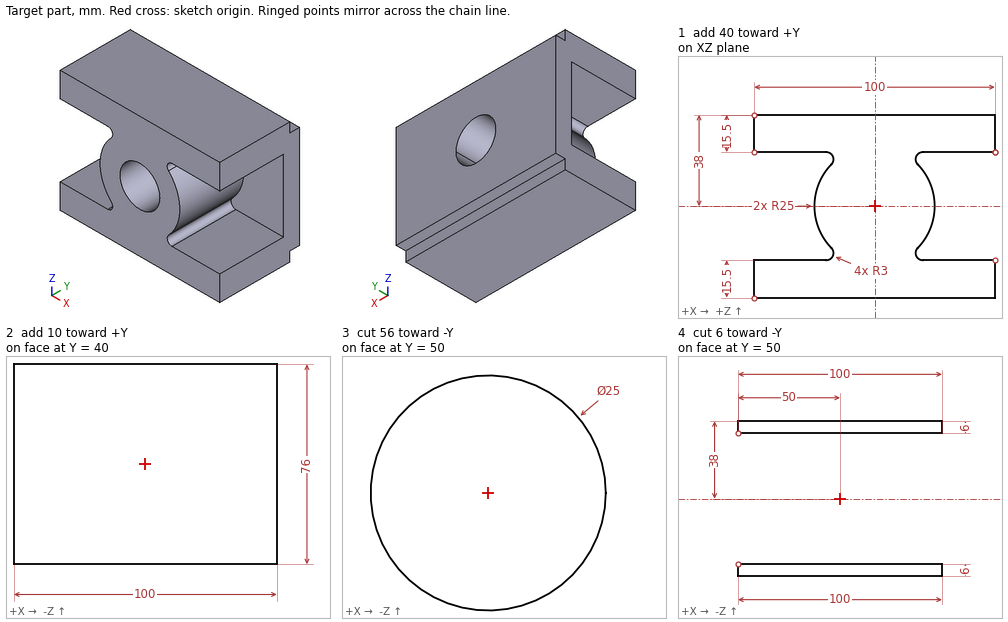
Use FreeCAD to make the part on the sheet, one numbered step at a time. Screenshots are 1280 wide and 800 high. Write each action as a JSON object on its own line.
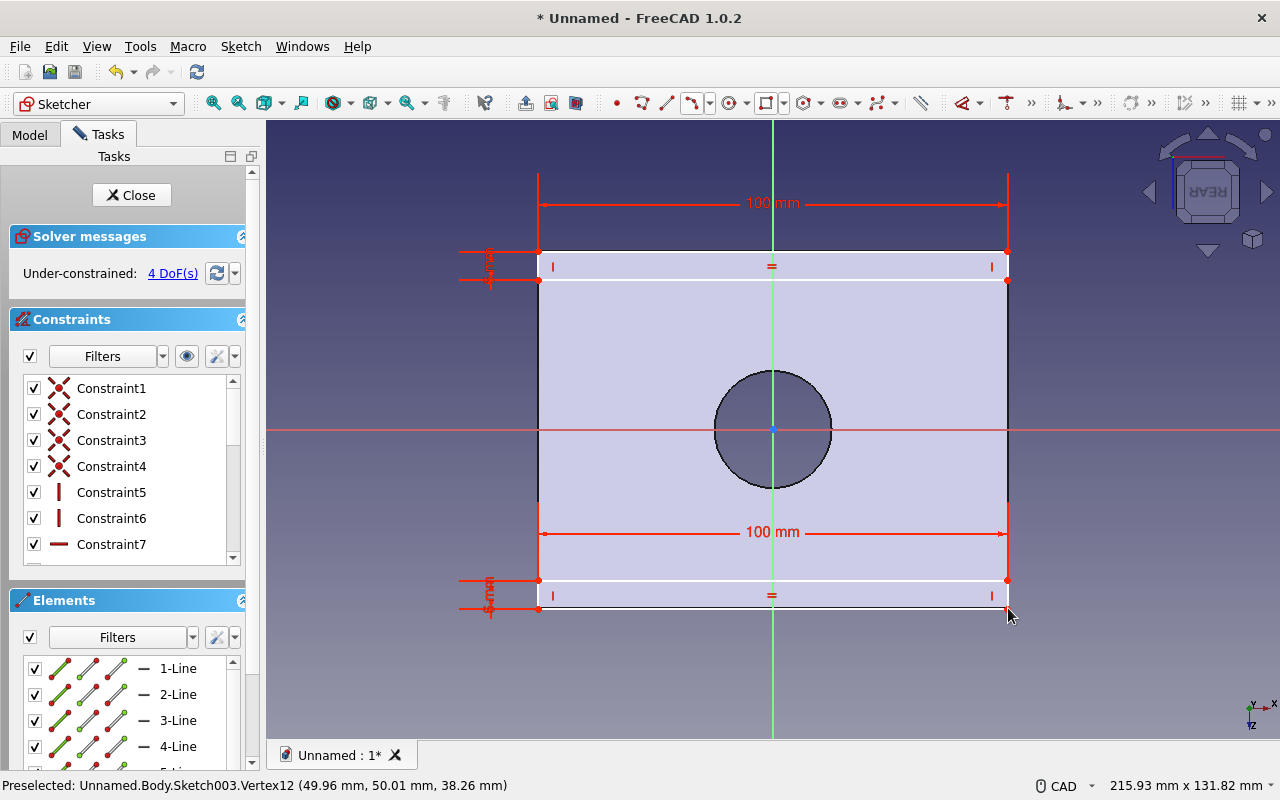
{"action": "left_click", "coordinate": [538, 280]}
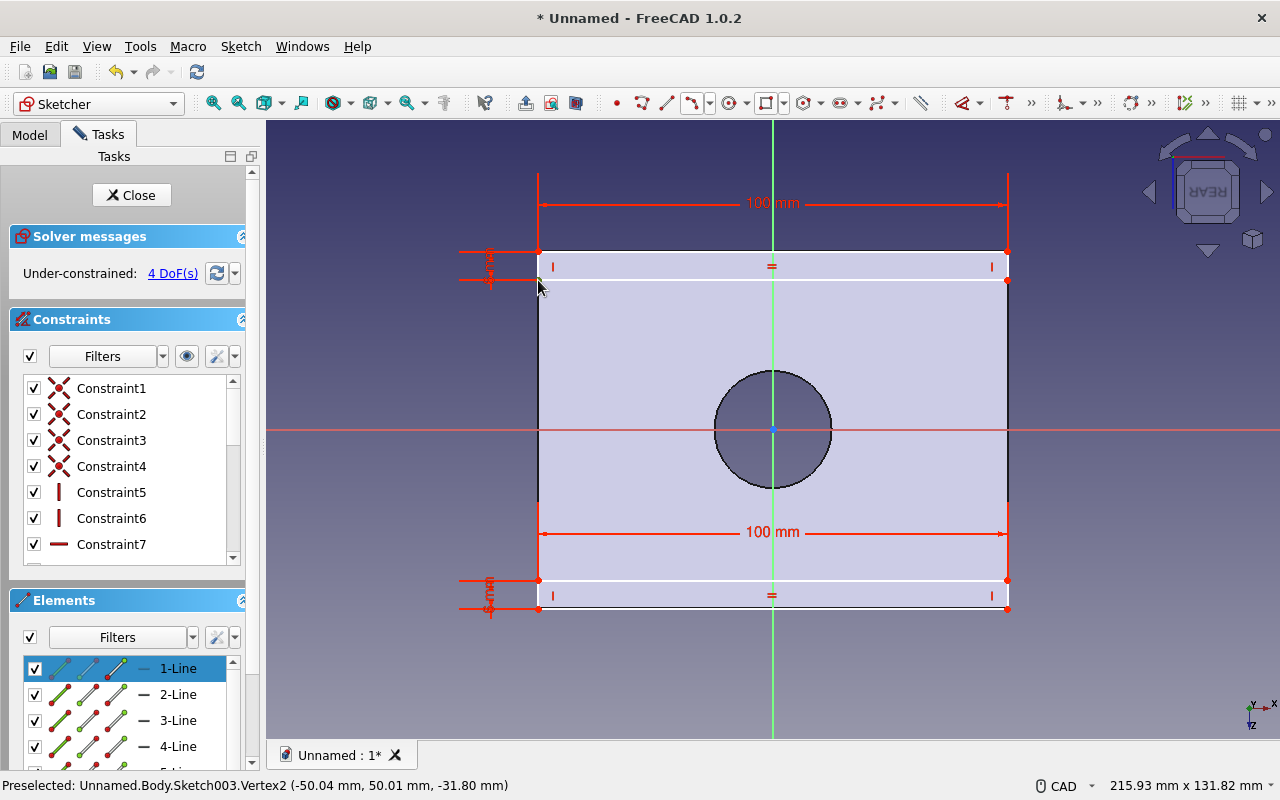
{"action": "left_click", "coordinate": [538, 581]}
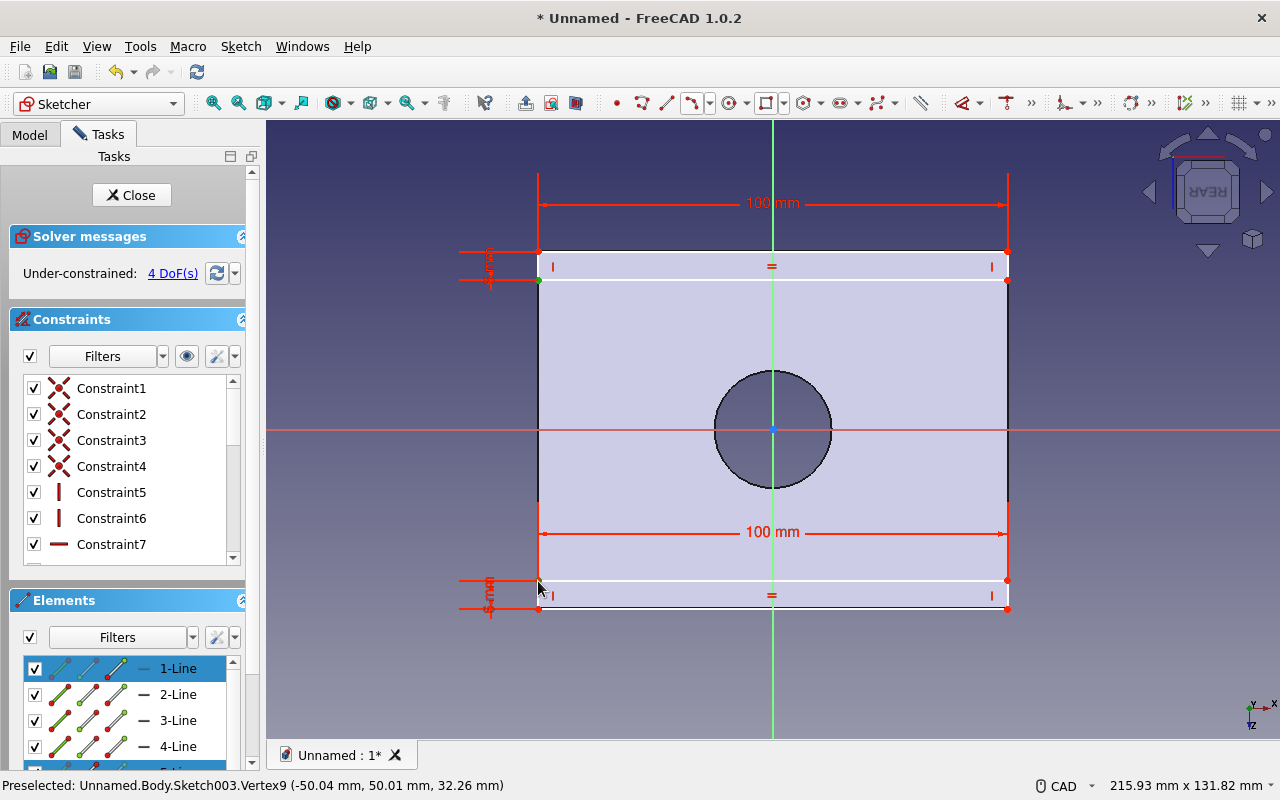
{"action": "left_click", "coordinate": [353, 429]}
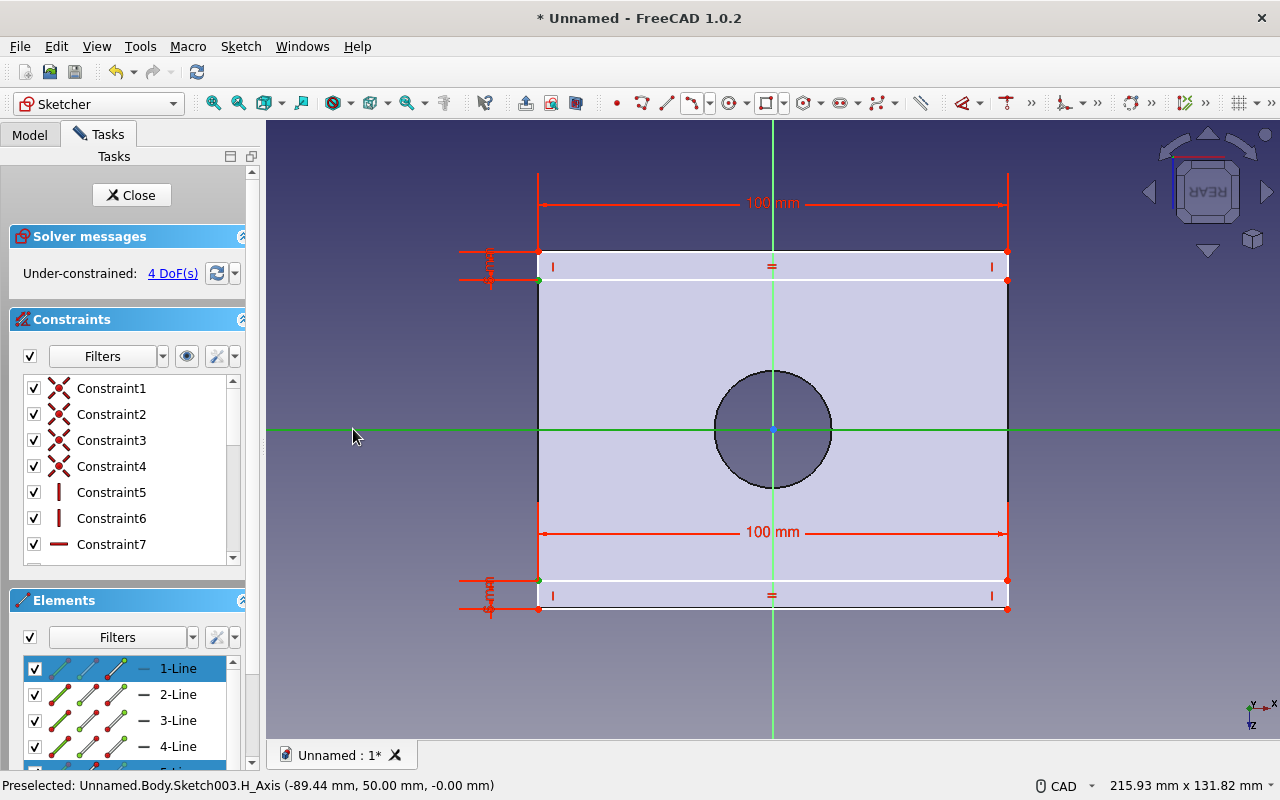
{"action": "key", "text": "s"}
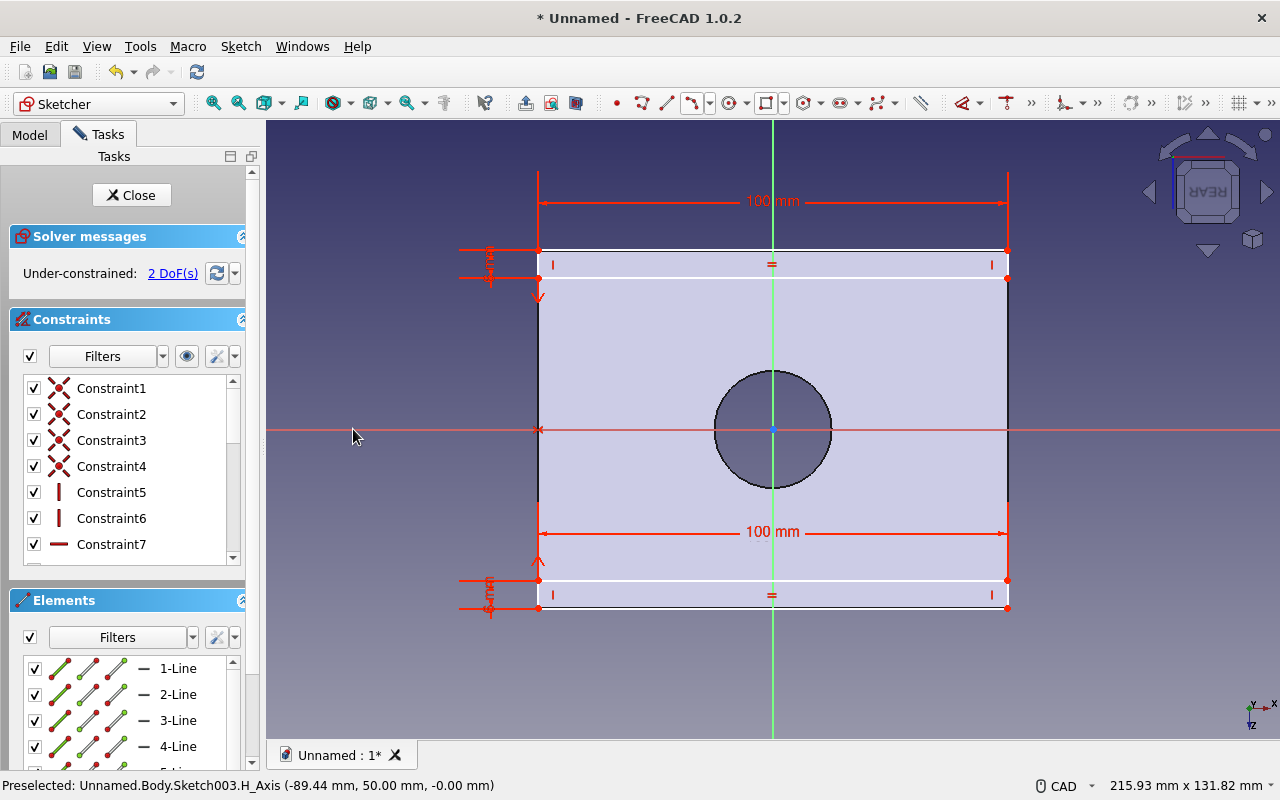
{"action": "left_click", "coordinate": [962, 104]}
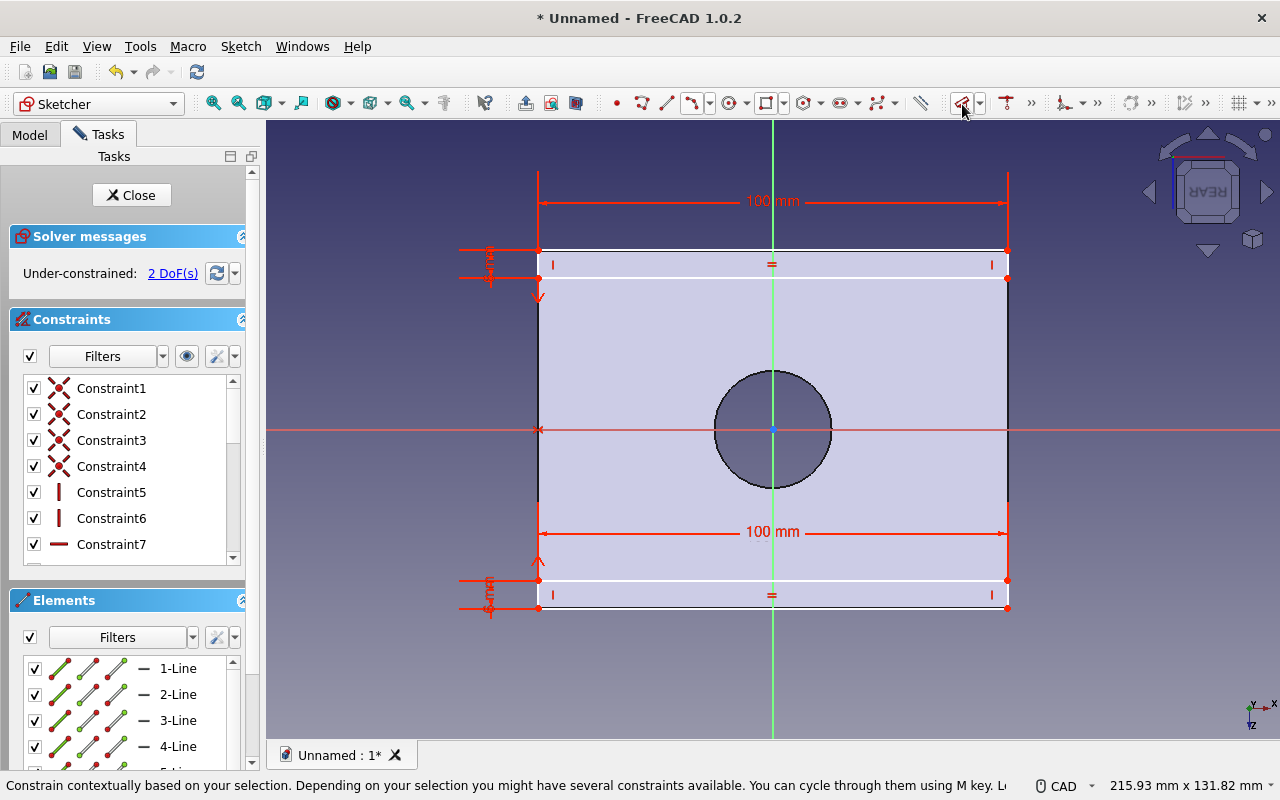
{"action": "left_click", "coordinate": [538, 250]}
{"action": "left_click", "coordinate": [655, 216]}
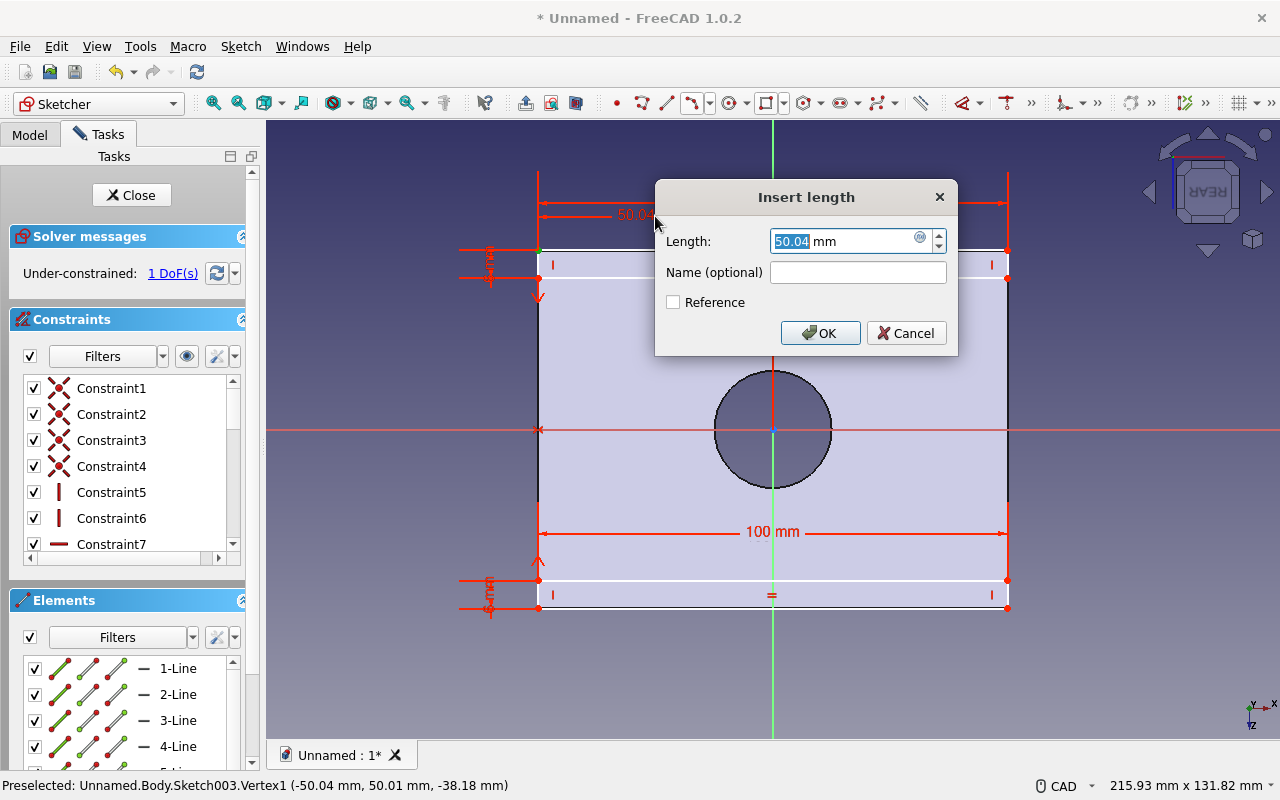
{"action": "type", "text": "50"}
{"action": "key", "text": "Return"}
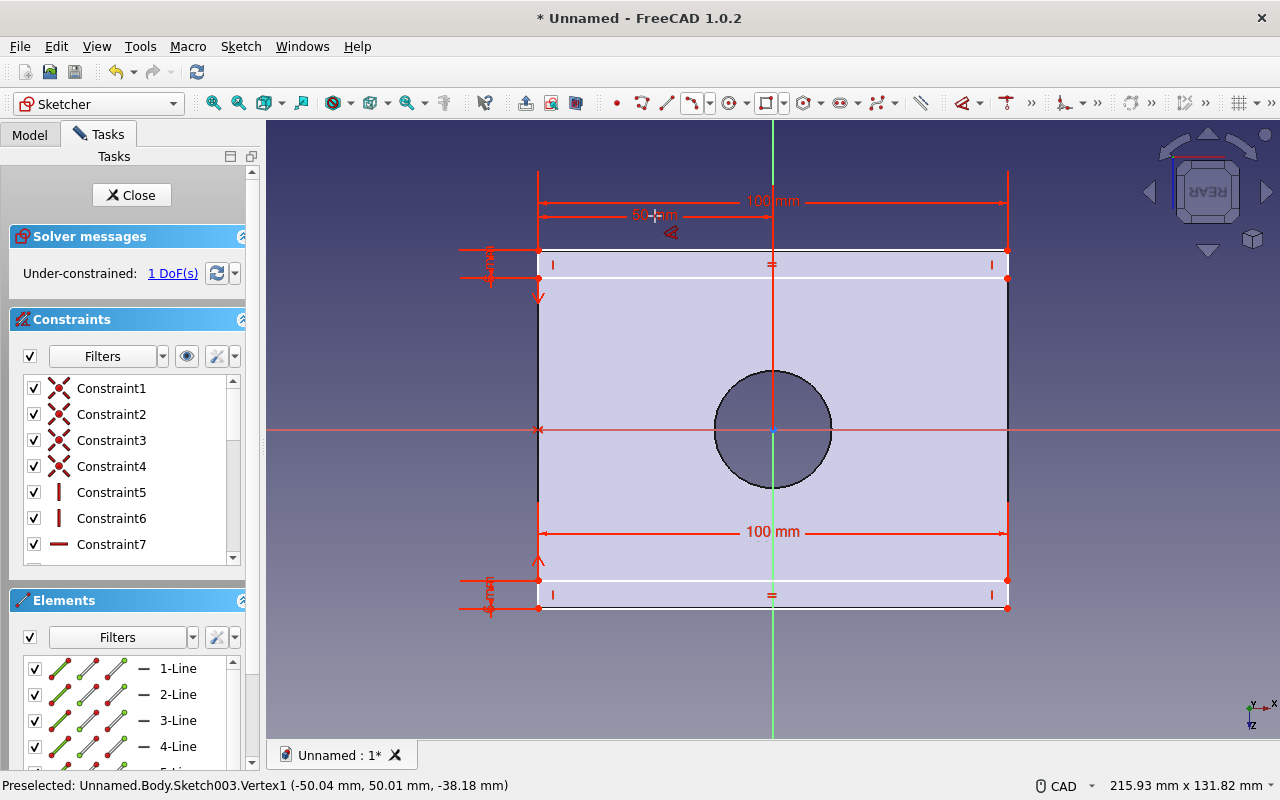
{"action": "left_click", "coordinate": [538, 250]}
{"action": "left_click", "coordinate": [504, 340]}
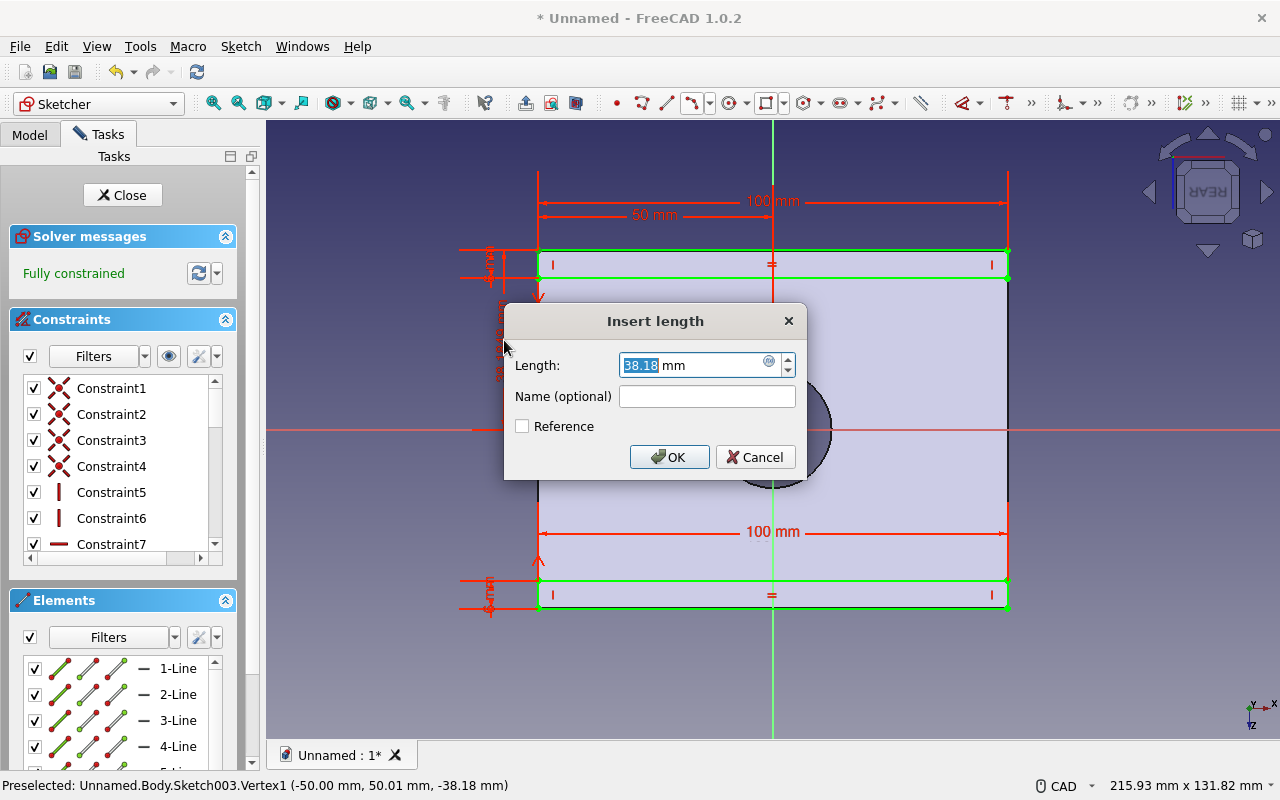
{"action": "type", "text": "38"}
{"action": "key", "text": "Return"}
{"action": "key", "text": "Escape"}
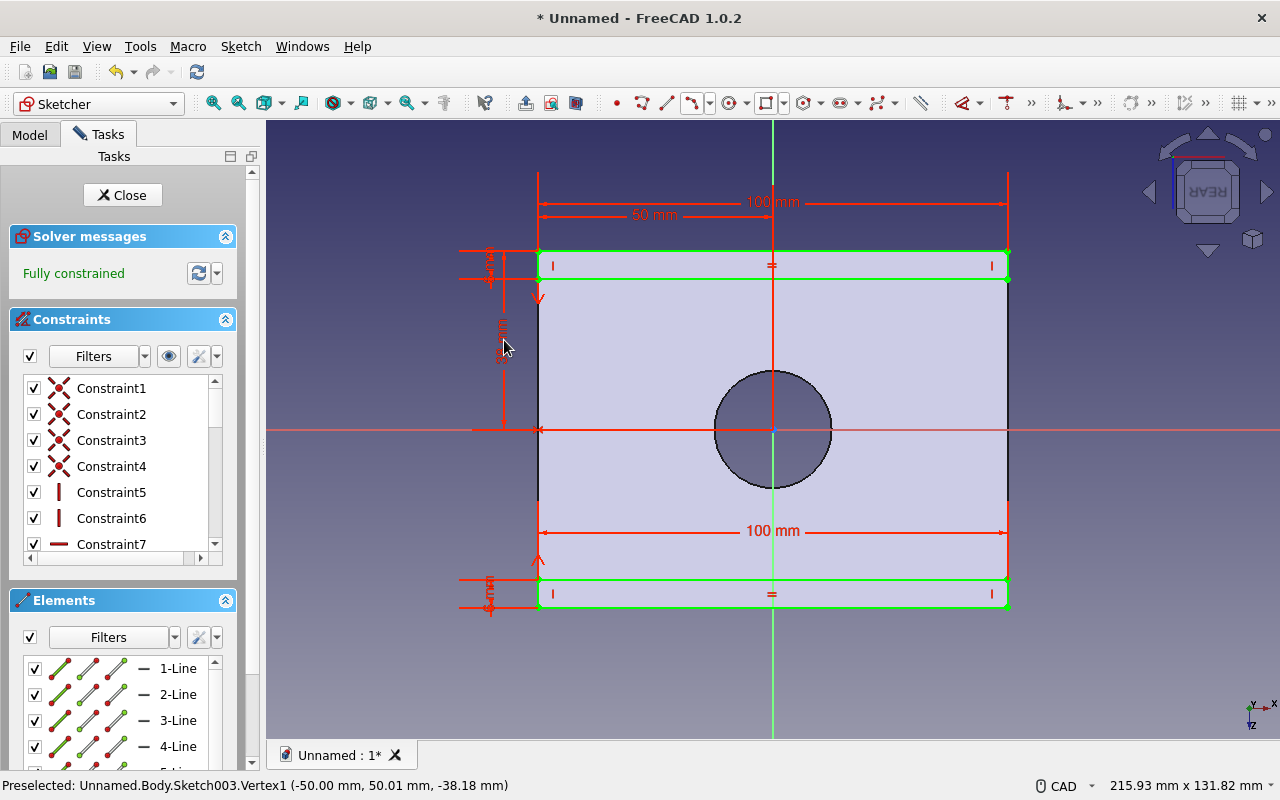
{"action": "left_click", "coordinate": [123, 195]}